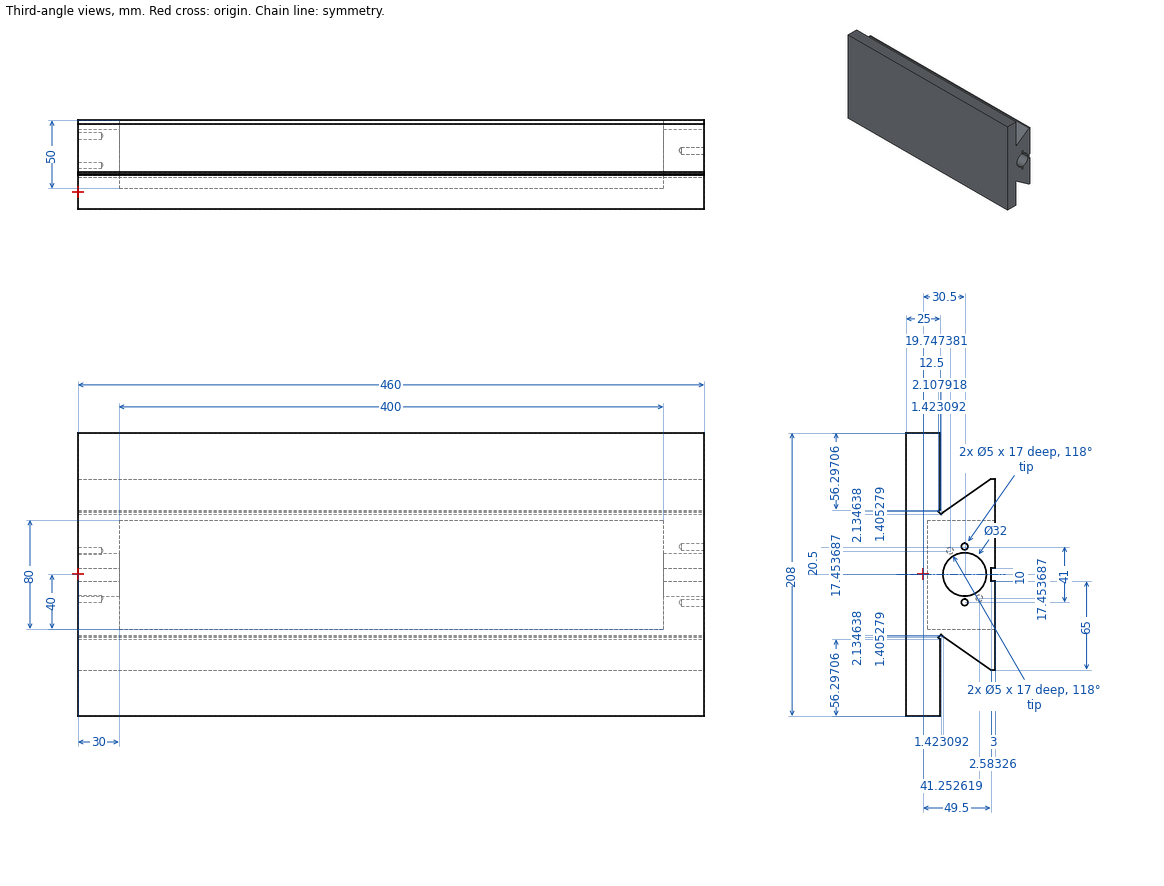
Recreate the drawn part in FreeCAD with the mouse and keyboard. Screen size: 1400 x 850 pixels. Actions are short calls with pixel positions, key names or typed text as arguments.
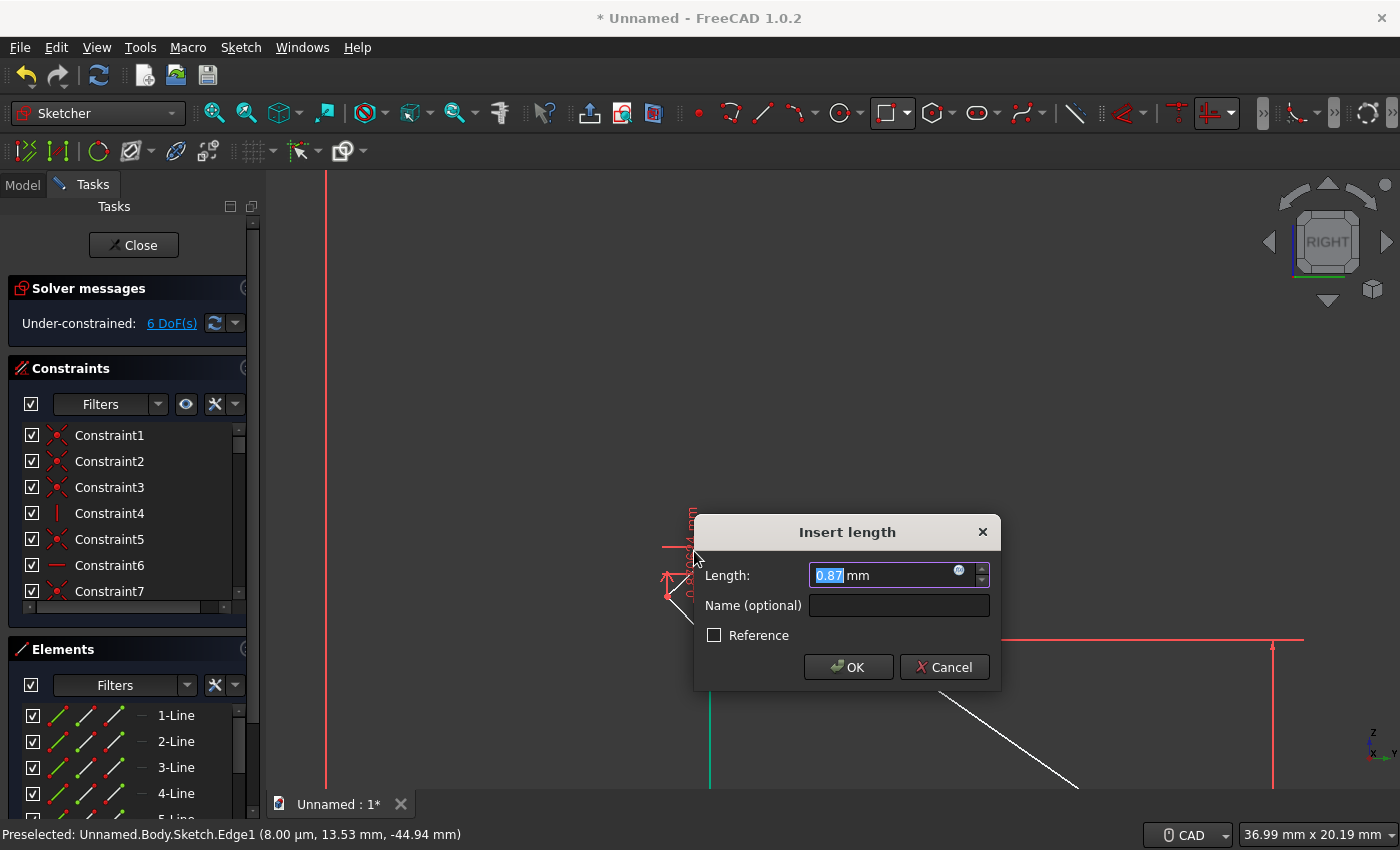
text(1.405279)
key(Return)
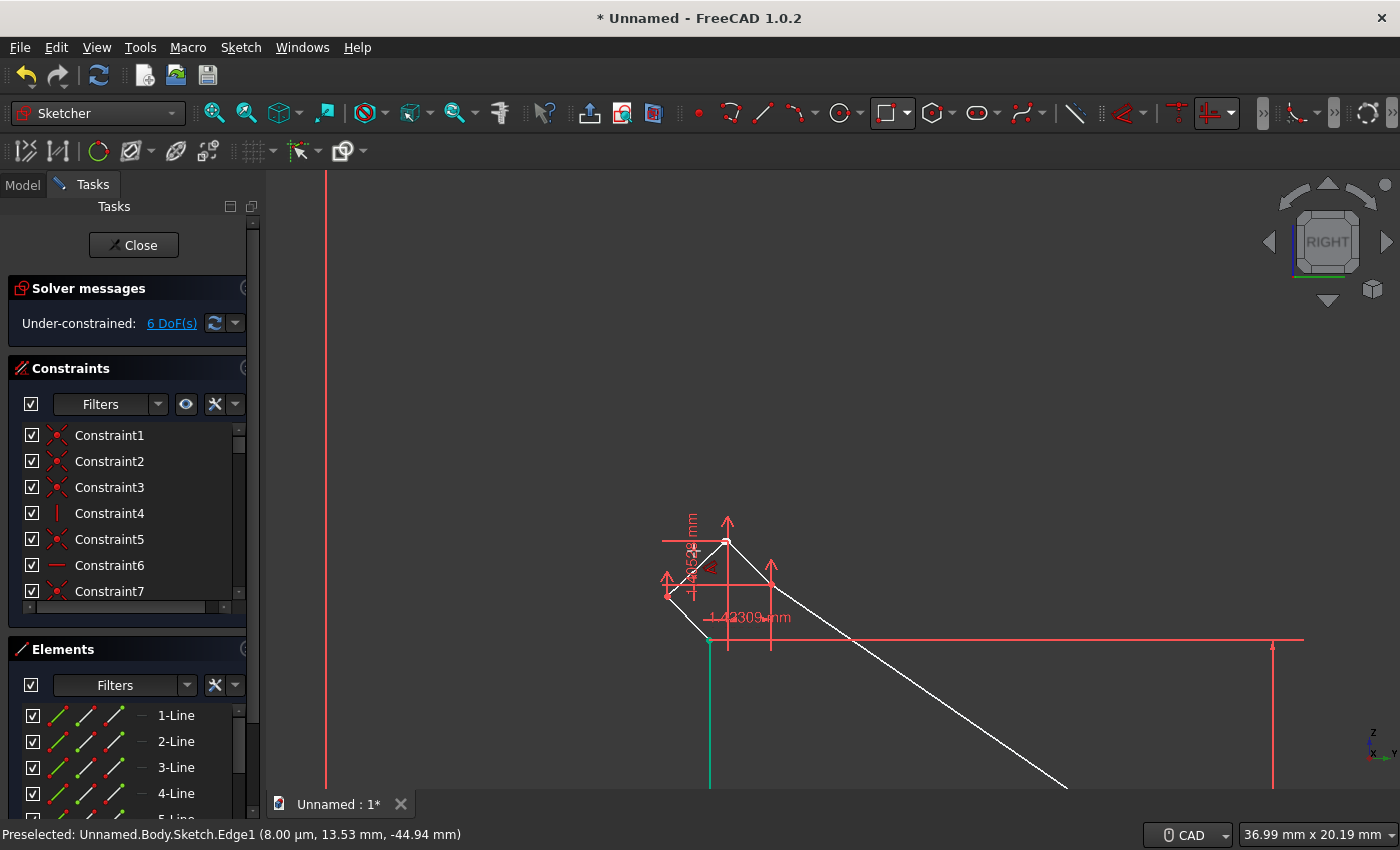
scroll(753, 564, down, 14)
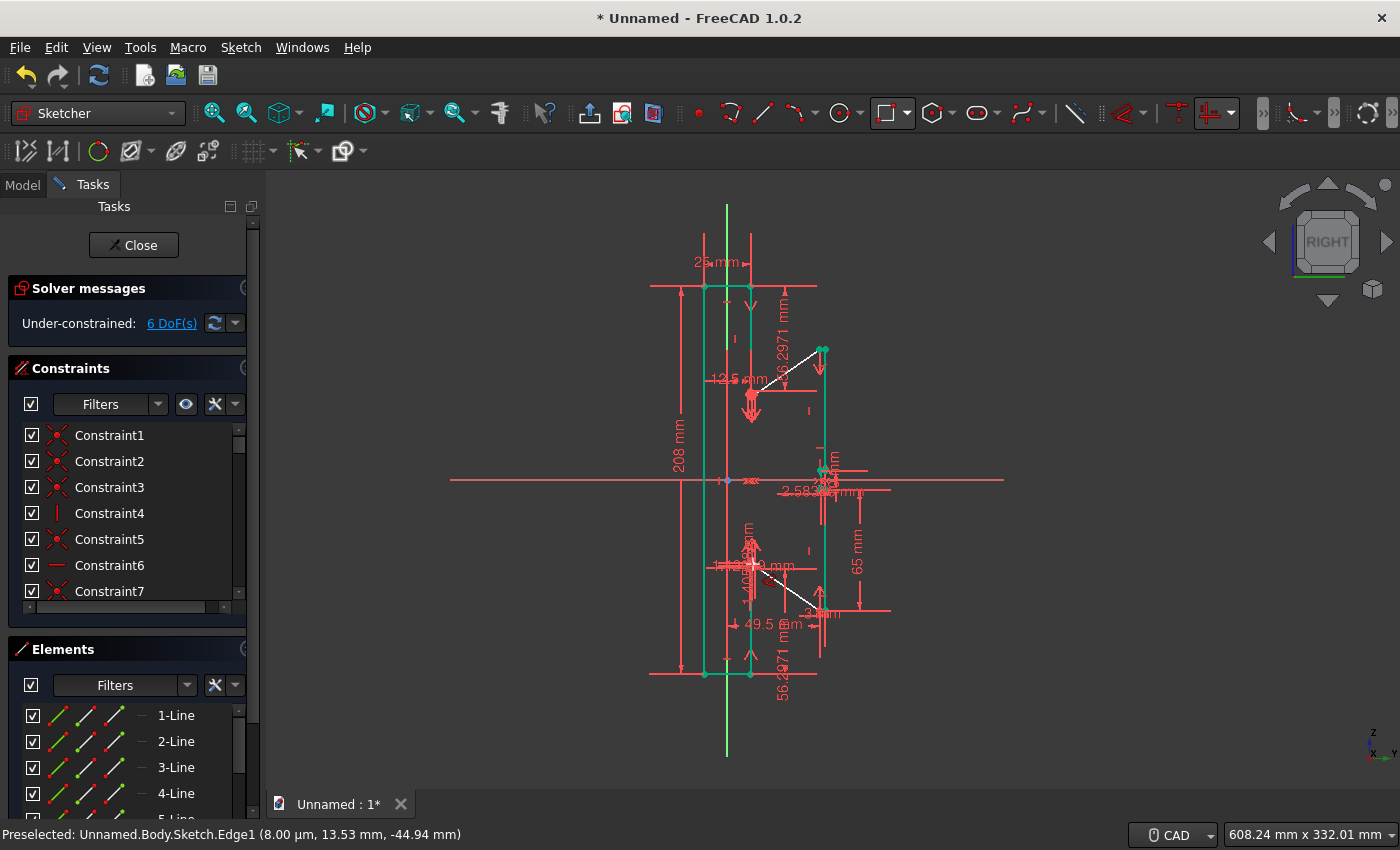
scroll(751, 396, up, 12)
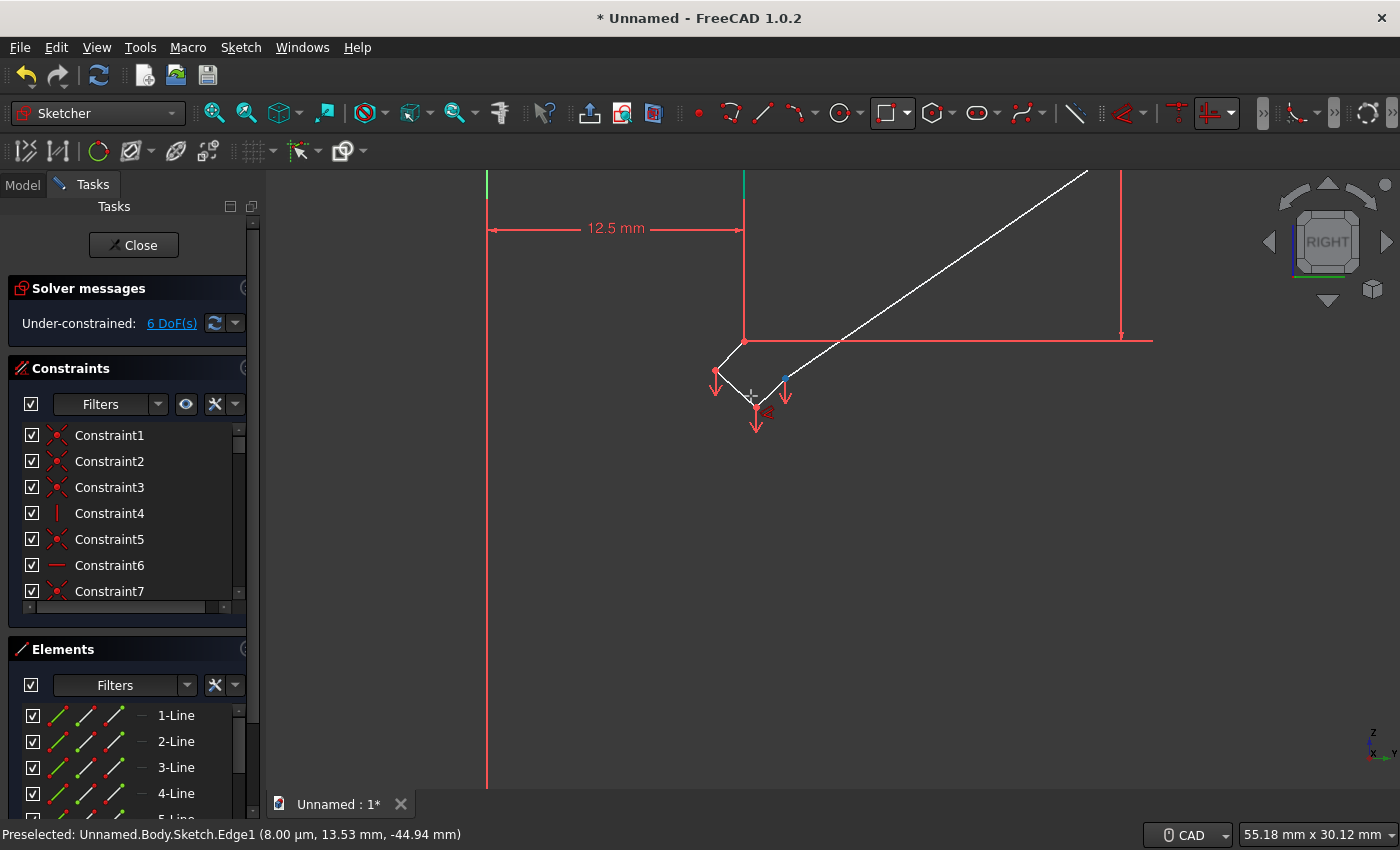
click(744, 397)
click(727, 337)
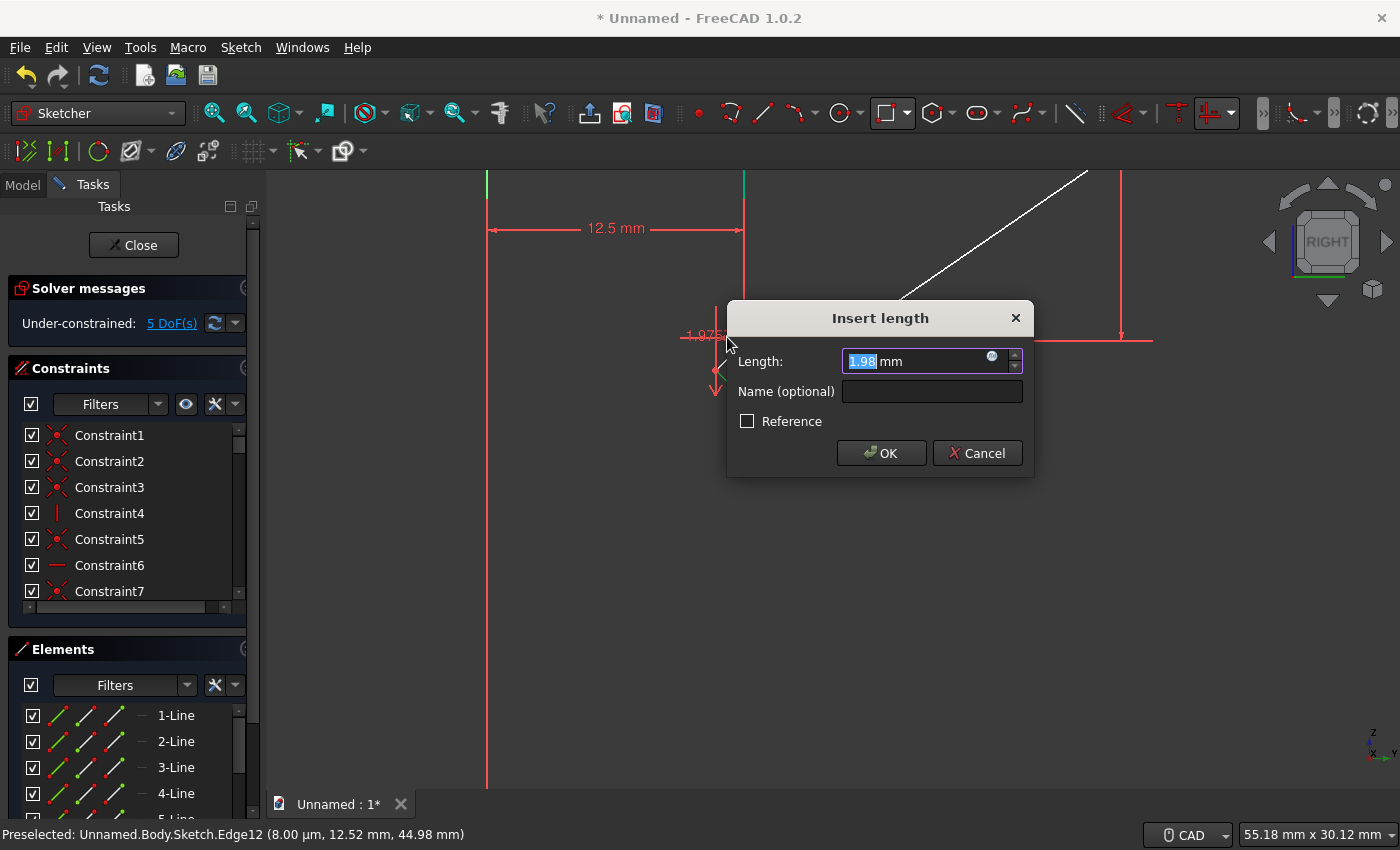
text(2.107918)
key(Return)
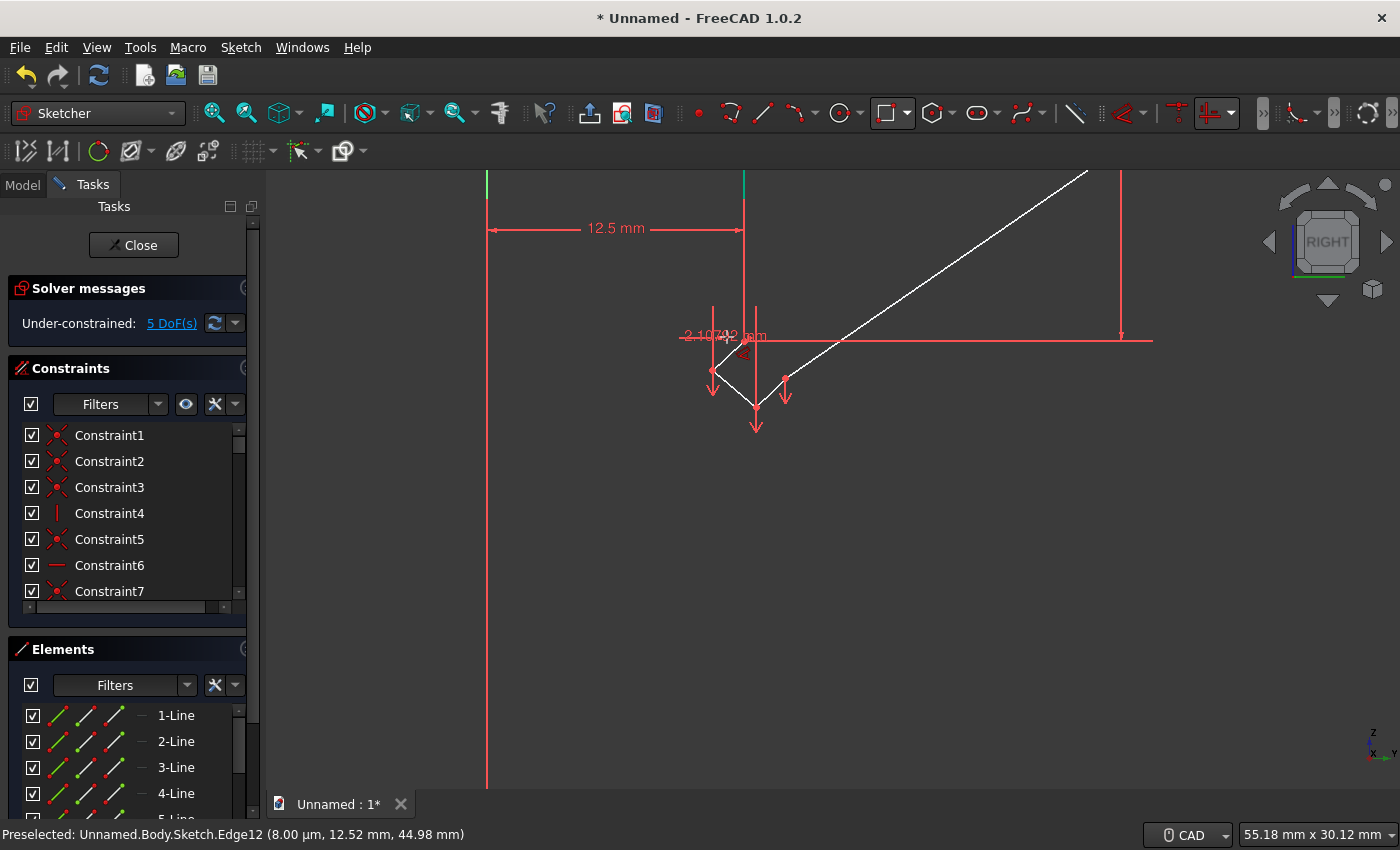
click(743, 397)
click(679, 389)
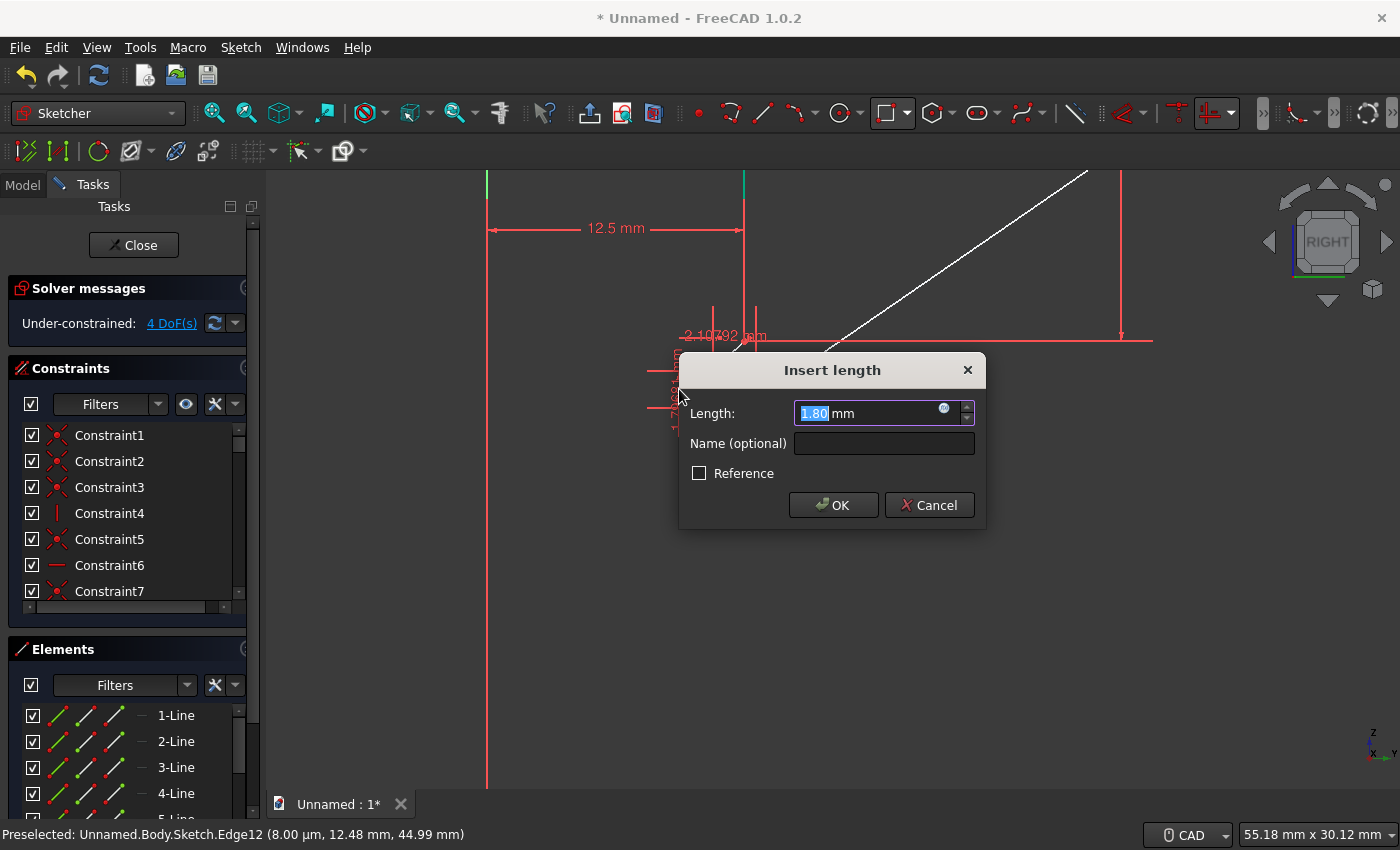
text(2.134638)
key(Return)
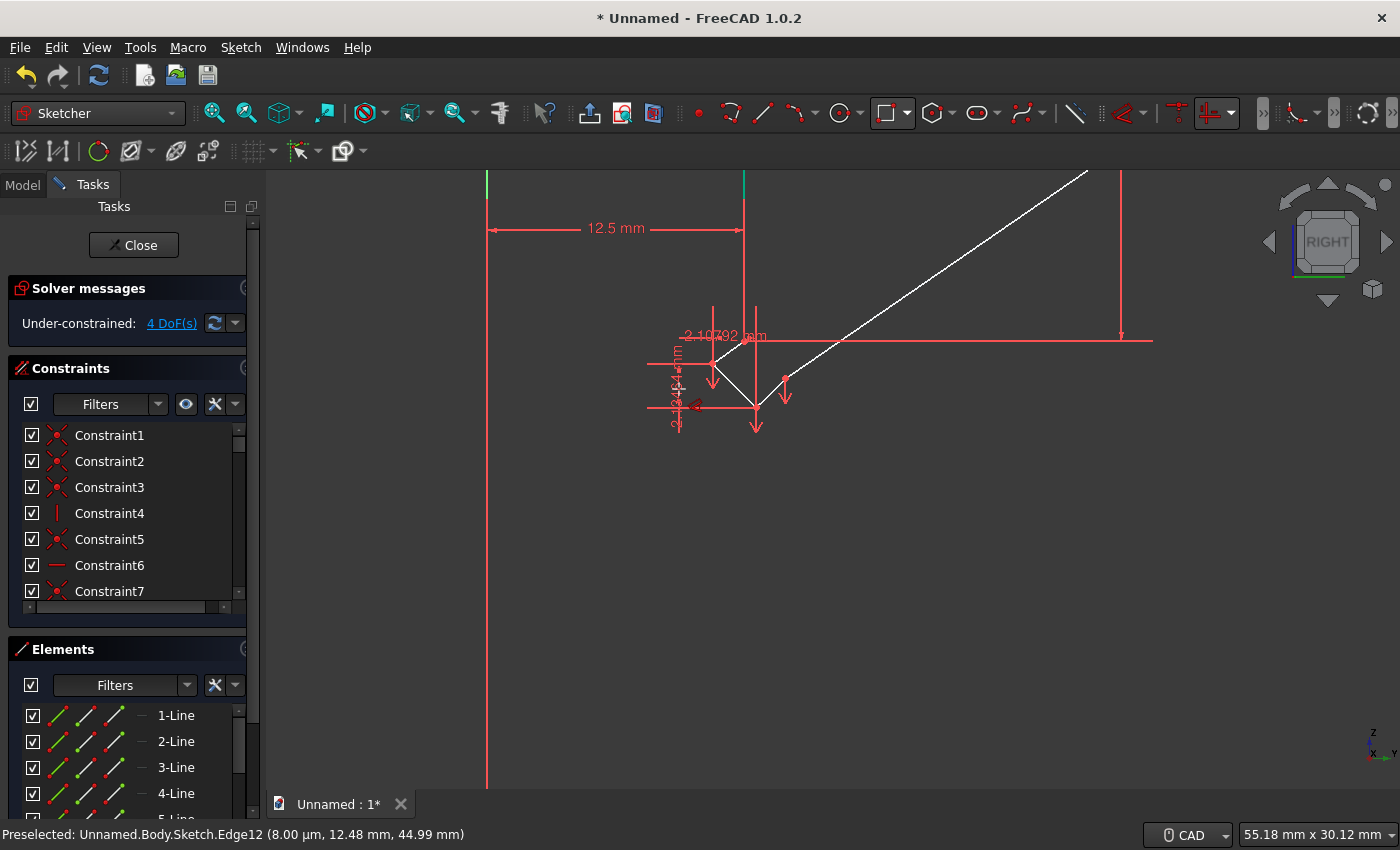
scroll(722, 357, up, 2)